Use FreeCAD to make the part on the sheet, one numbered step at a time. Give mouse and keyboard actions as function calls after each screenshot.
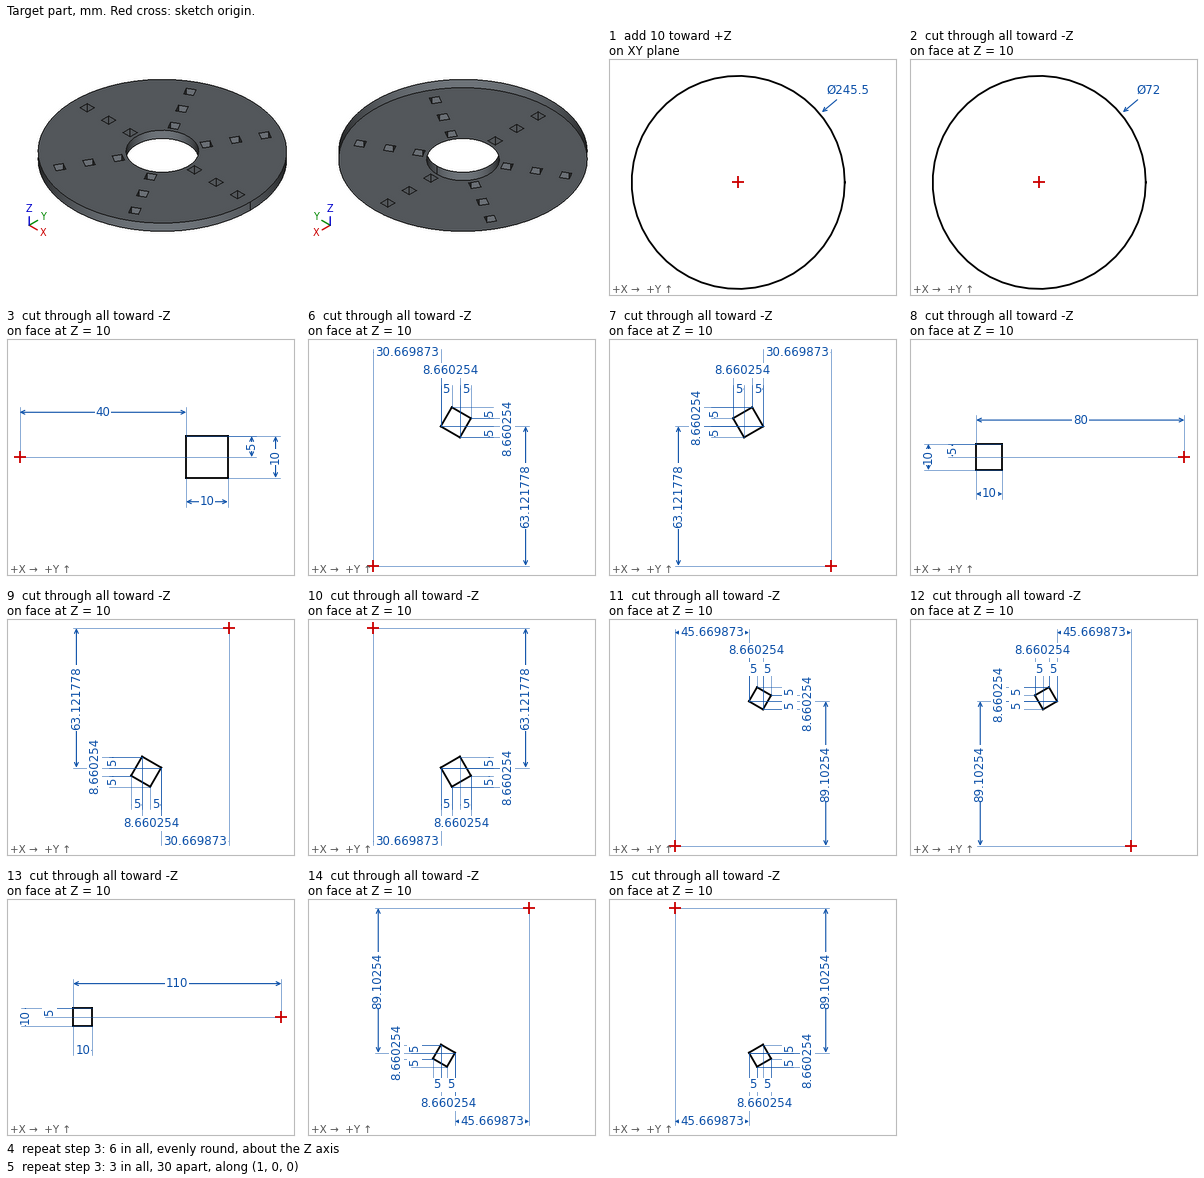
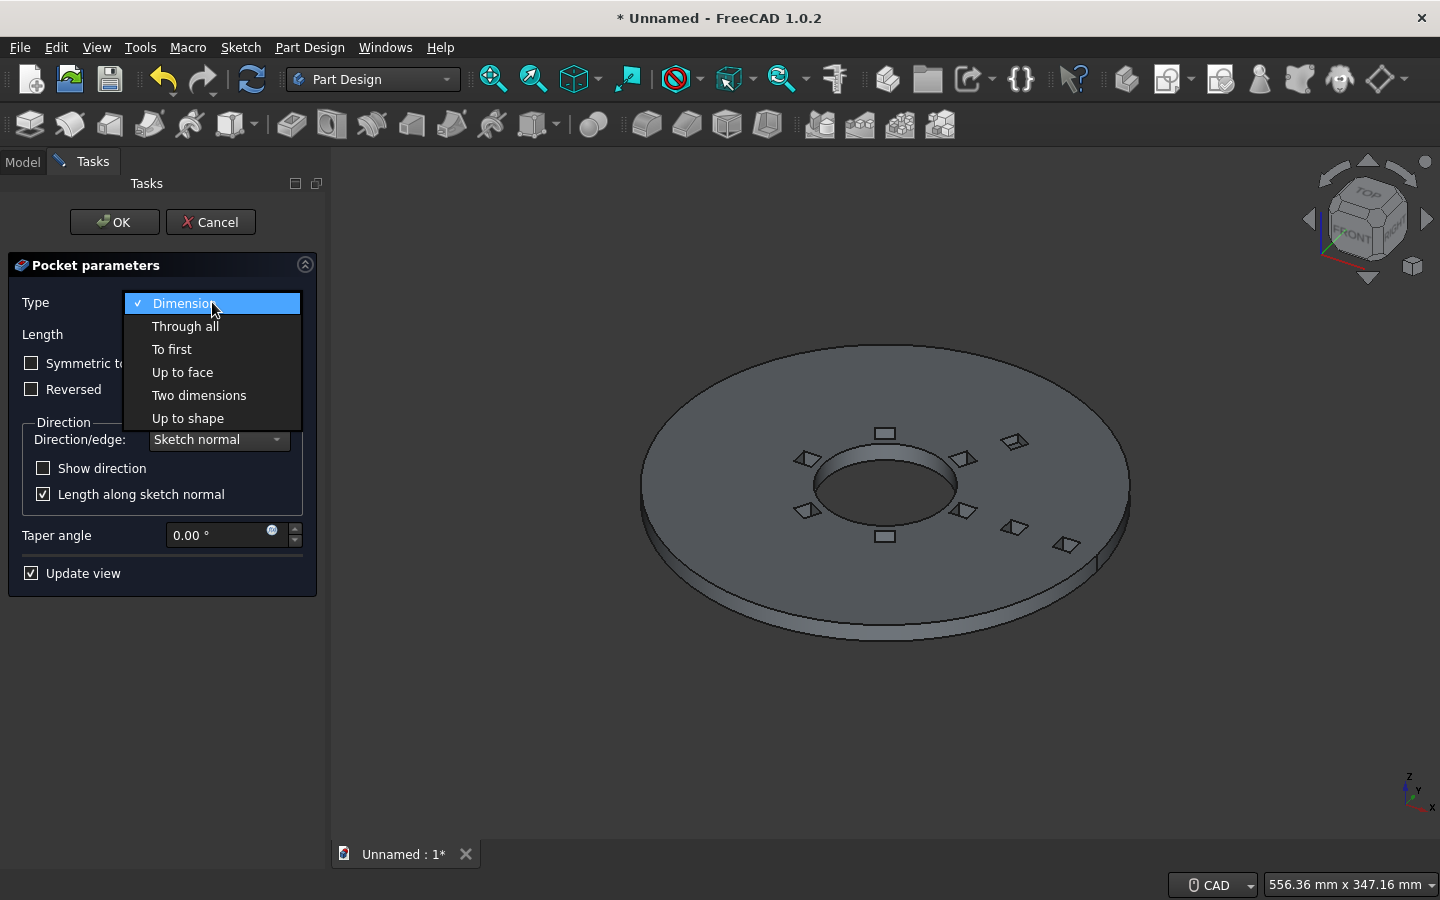
click(212, 326)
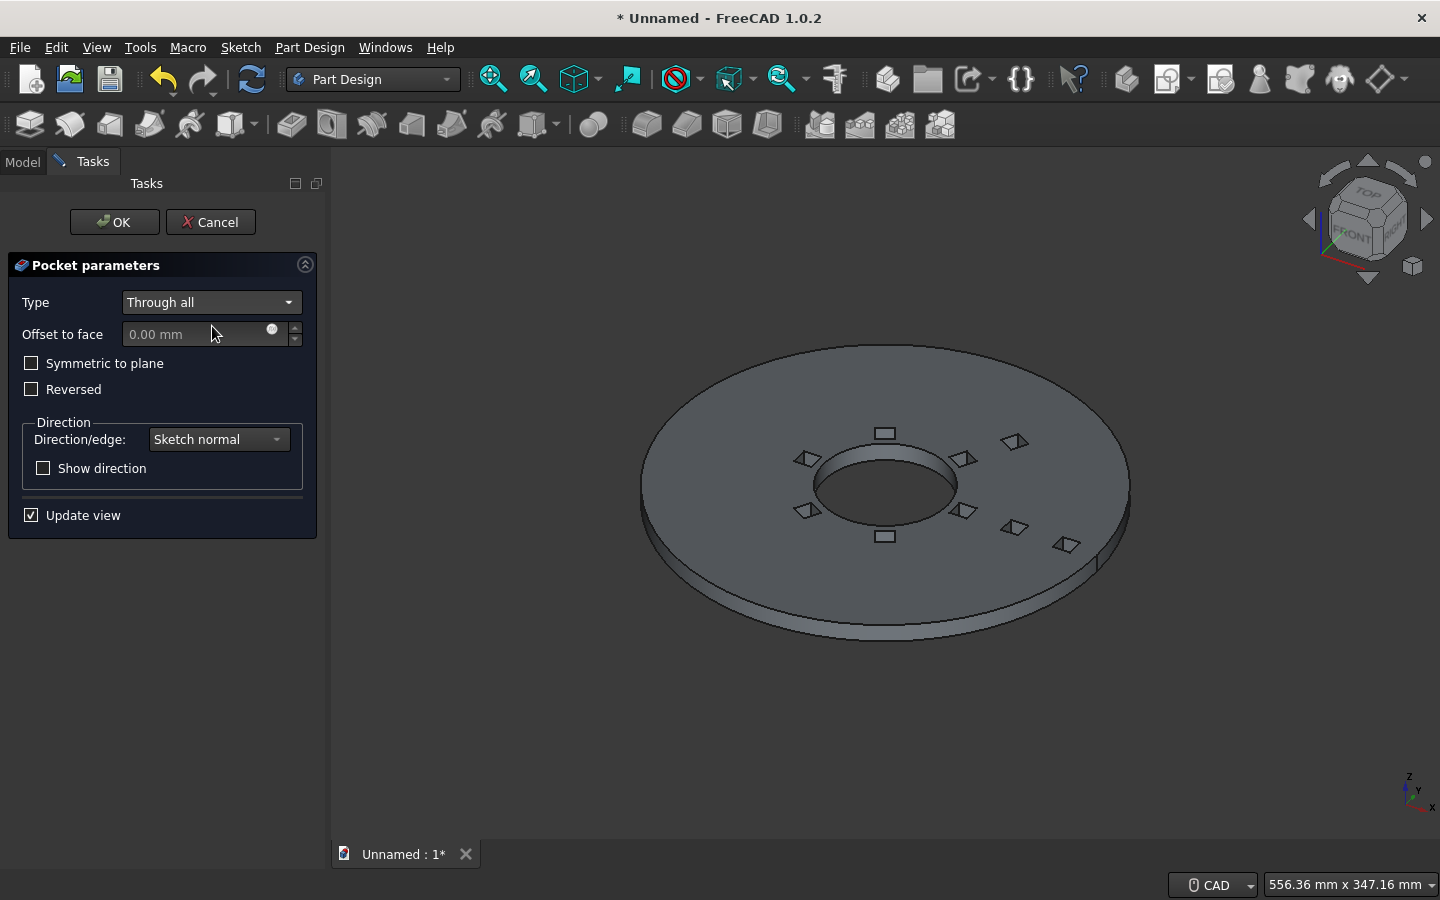
click(115, 222)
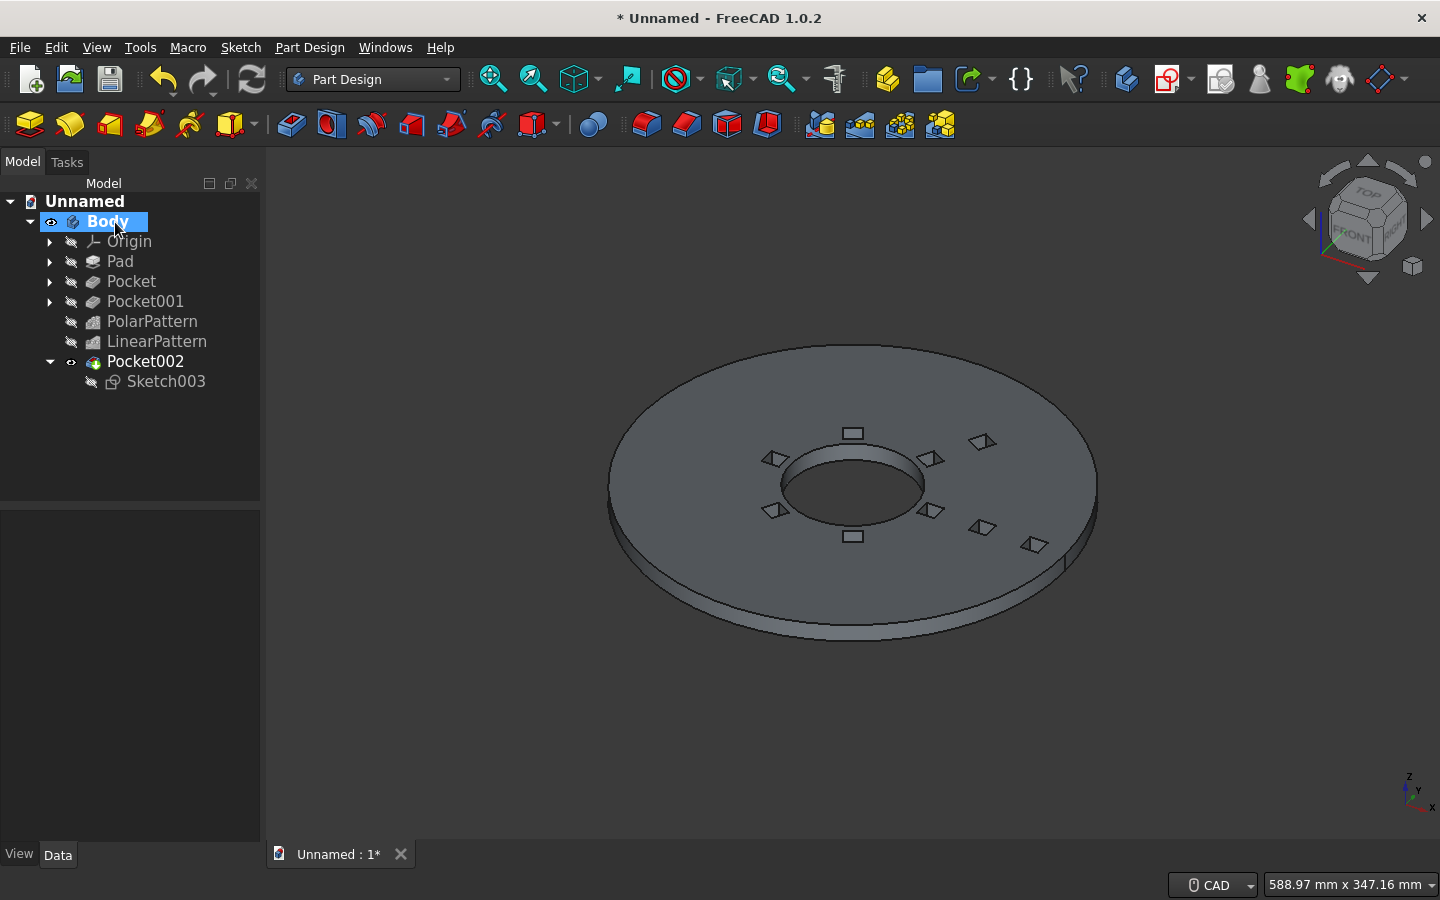
click(767, 409)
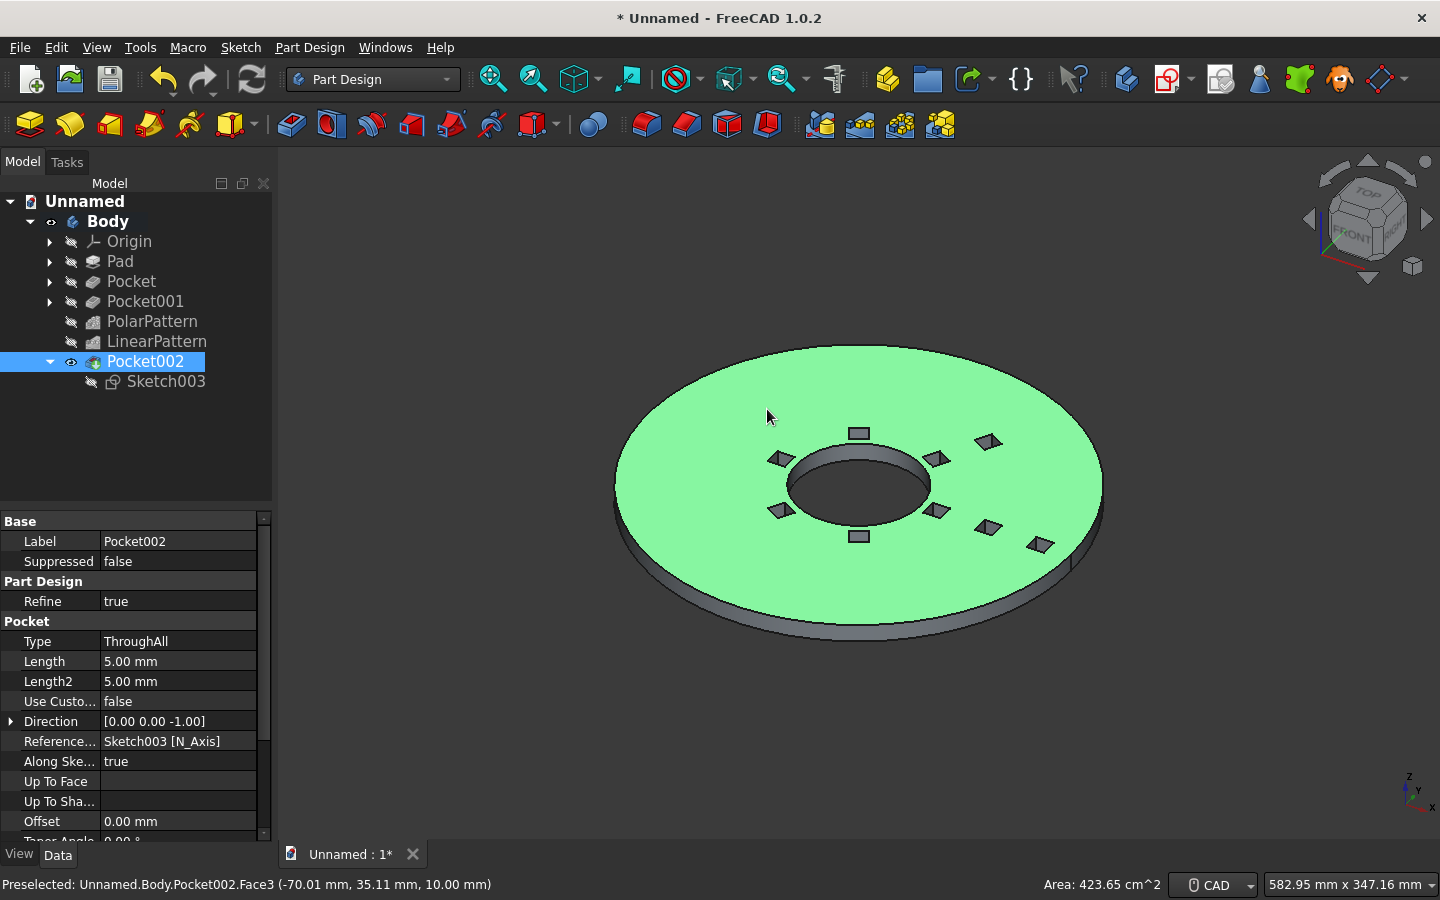
click(1168, 80)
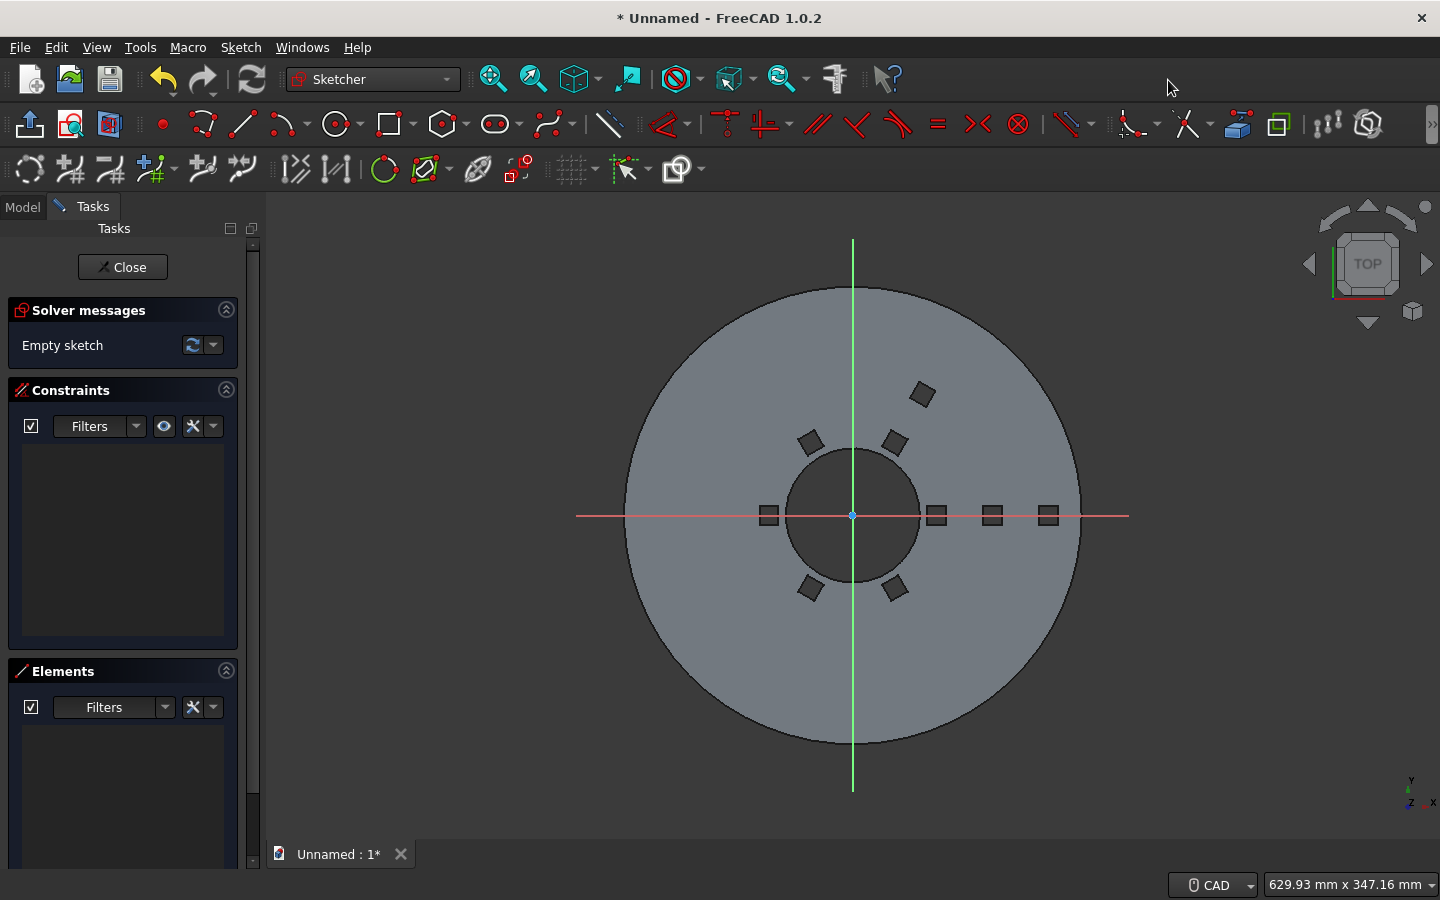
scroll(783, 387, up, 14)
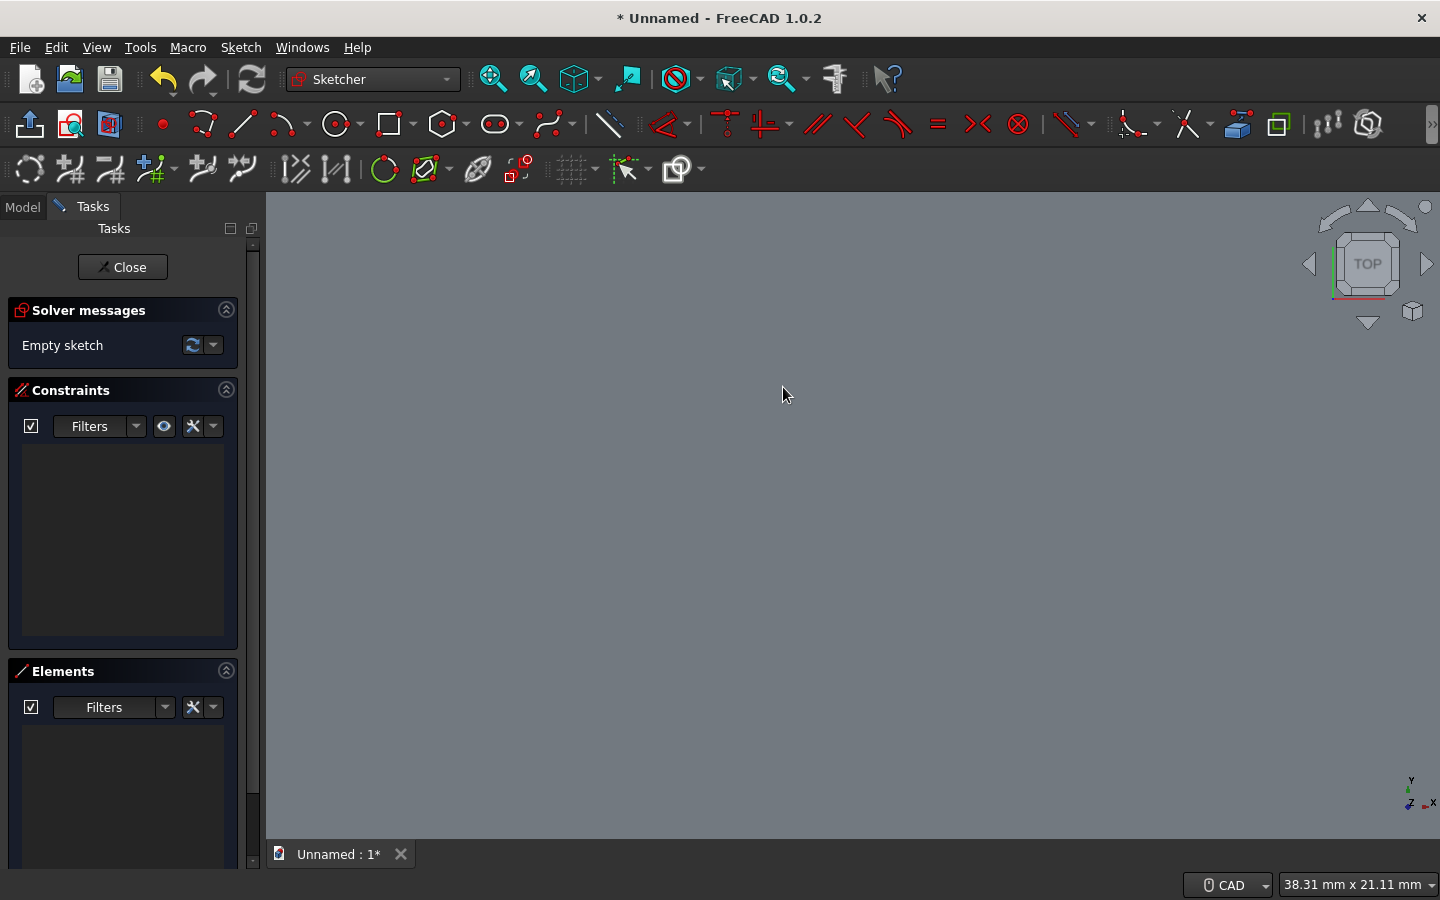
key(g)
key(m)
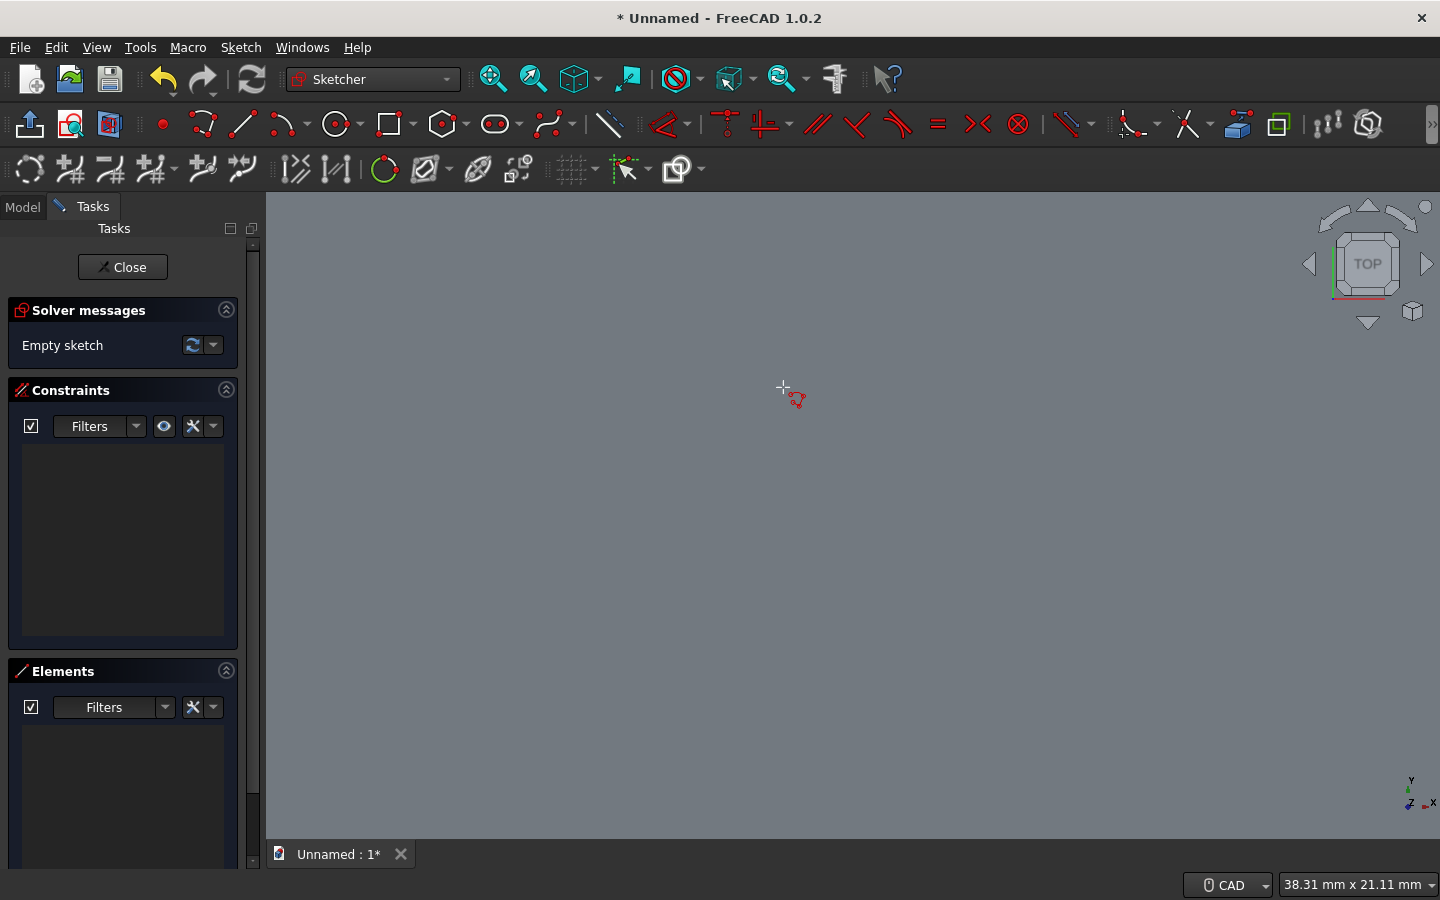
click(985, 561)
click(832, 296)
click(566, 449)
click(719, 714)
click(985, 562)
key(Escape)
key(Escape)